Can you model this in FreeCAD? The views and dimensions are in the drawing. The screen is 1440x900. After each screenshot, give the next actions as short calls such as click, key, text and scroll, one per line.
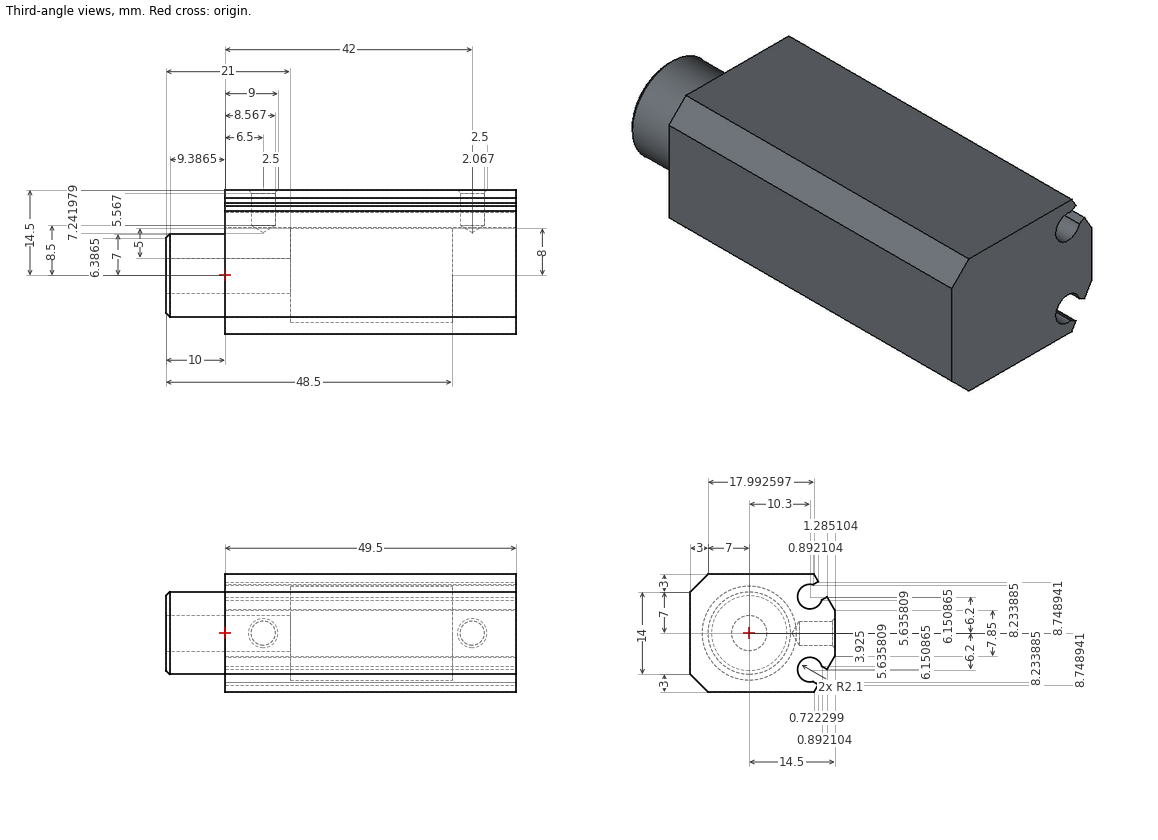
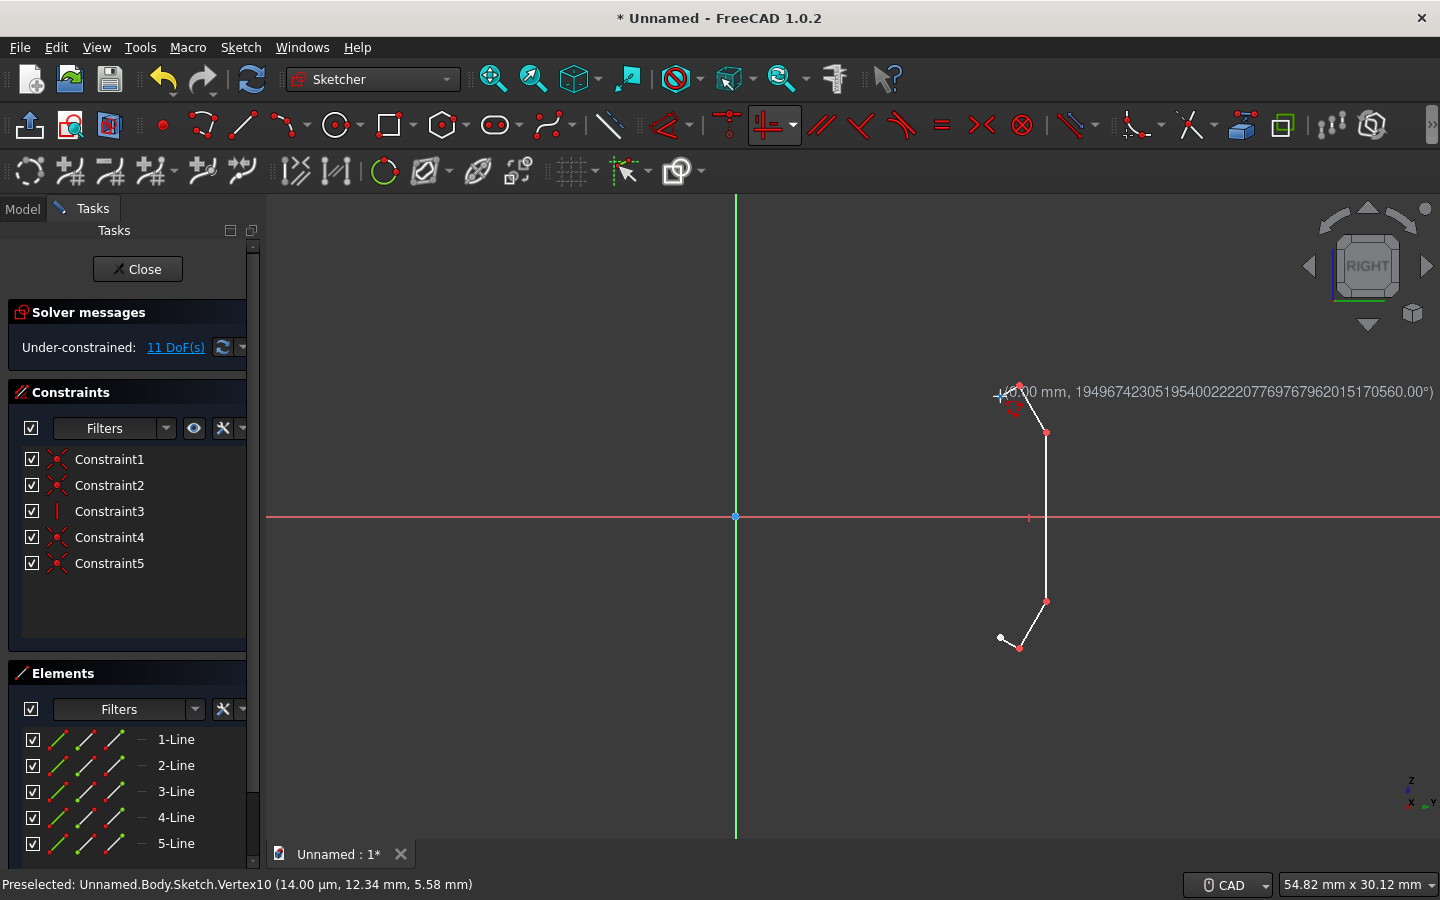
click(968, 340)
click(987, 329)
click(971, 302)
click(586, 302)
click(522, 367)
click(522, 666)
click(586, 731)
click(971, 731)
click(987, 704)
click(968, 693)
right_click(968, 693)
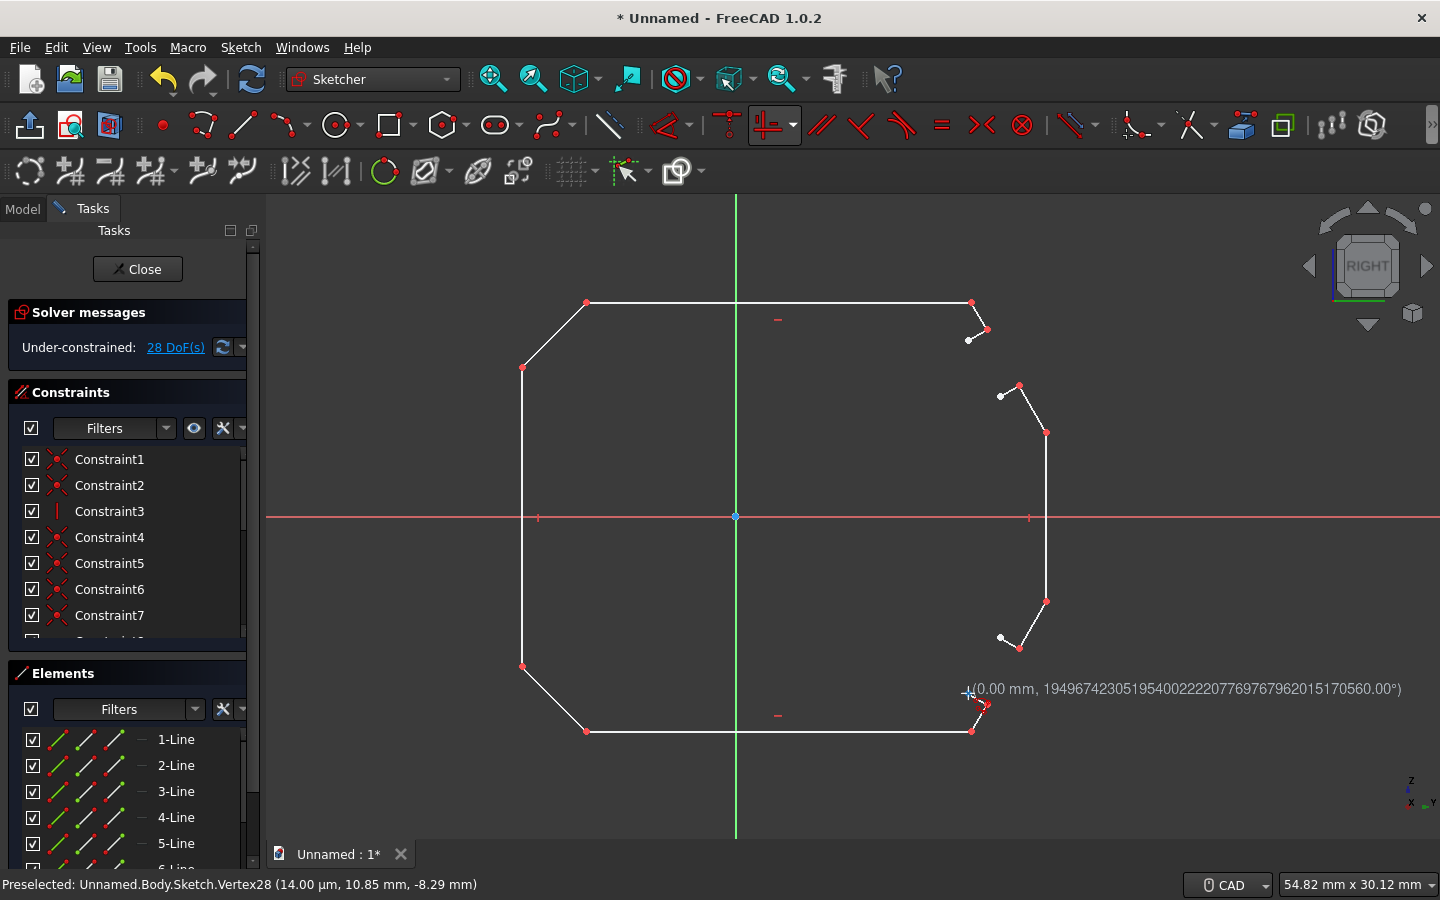
key(g)
key(3)
key(a)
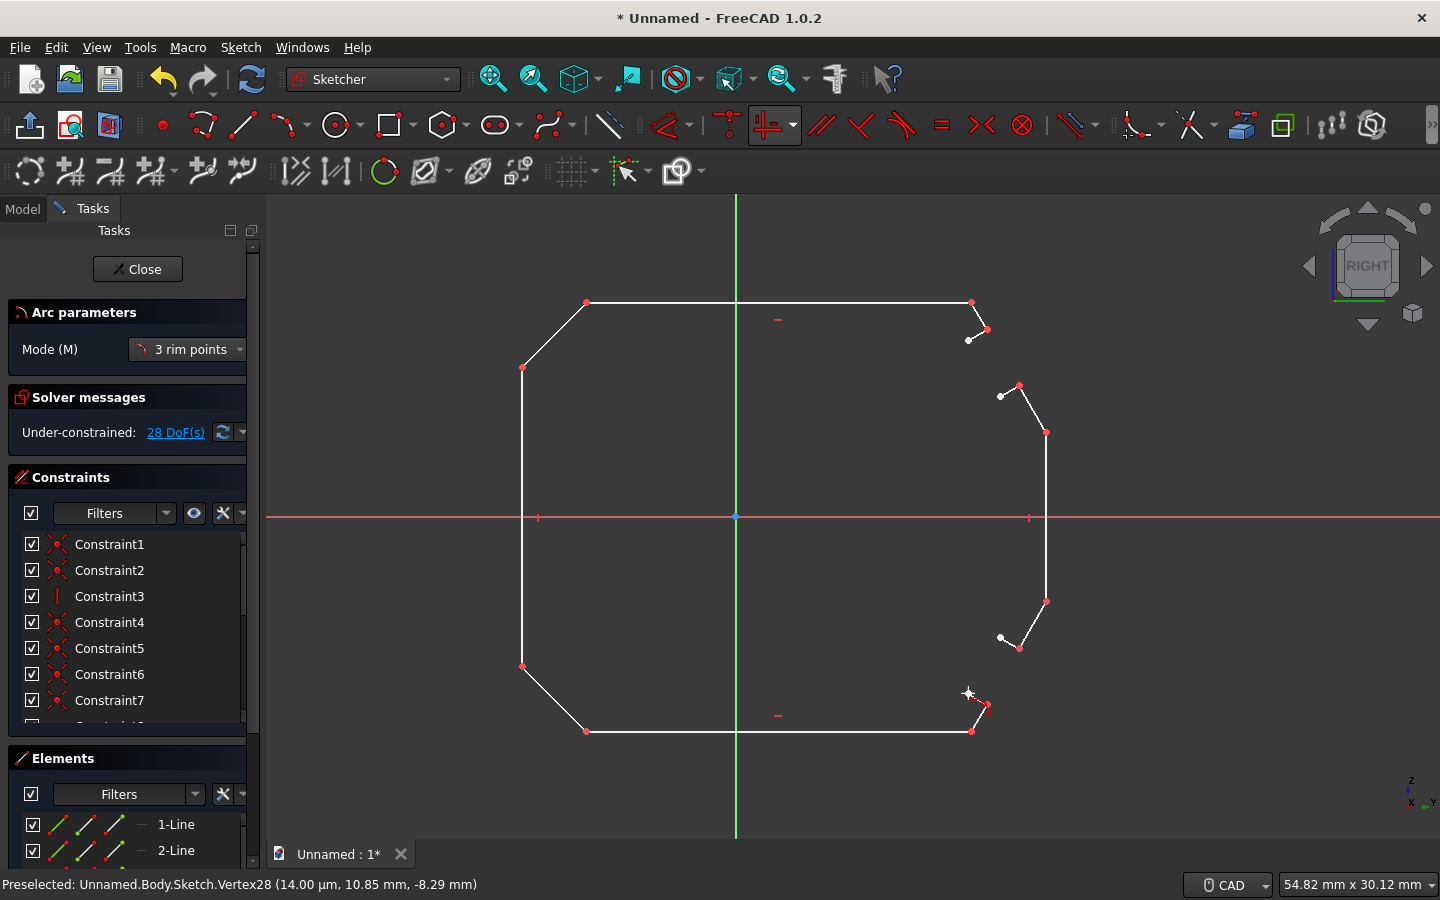
scroll(1000, 396, up, 2)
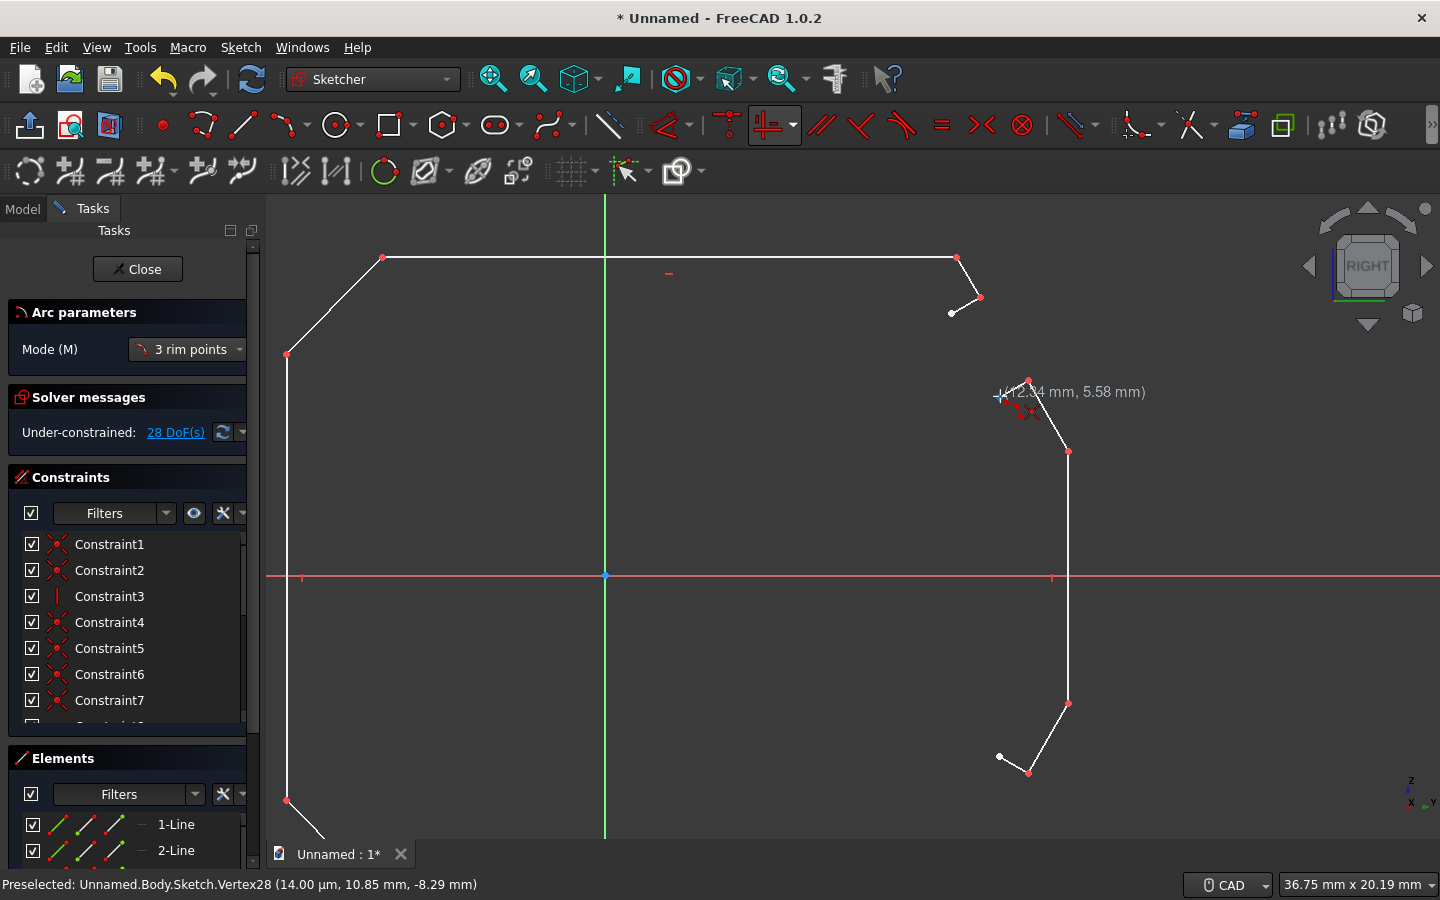
click(1000, 397)
click(952, 314)
click(876, 411)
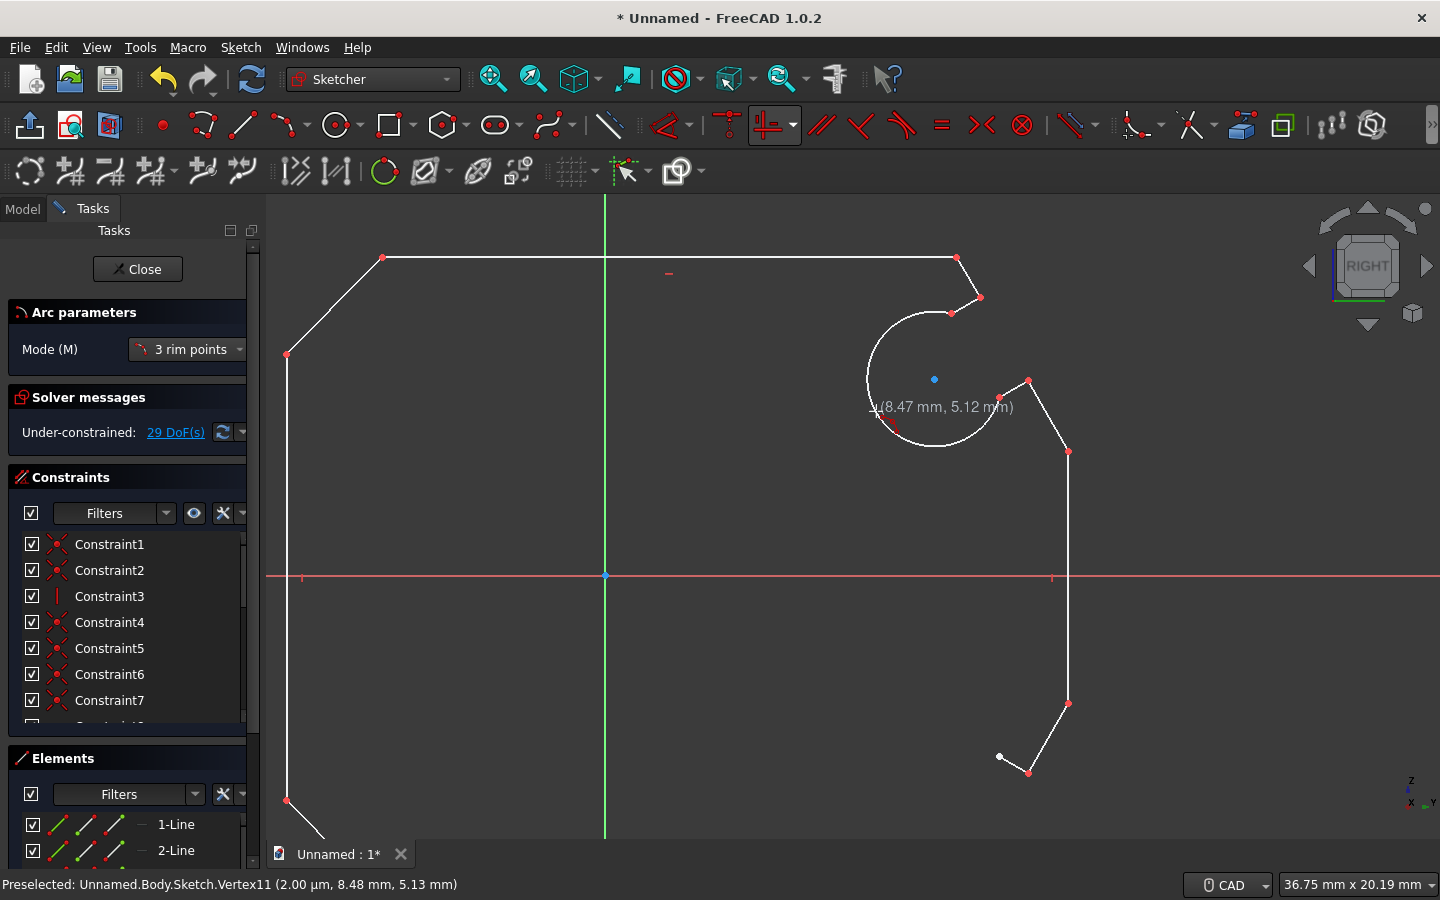
scroll(1002, 396, down, 2)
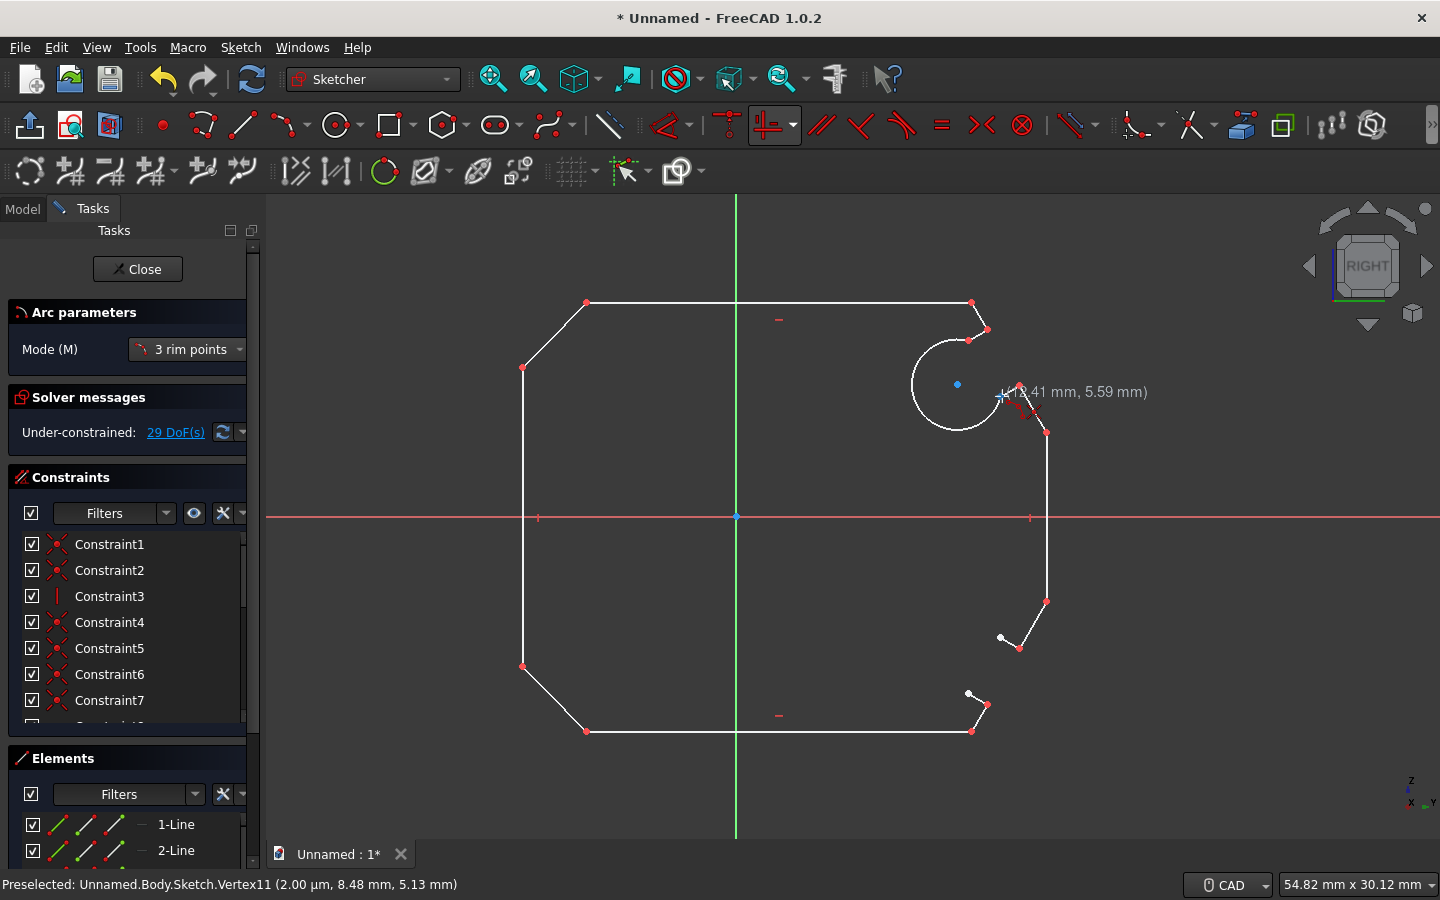
scroll(968, 693, up, 2)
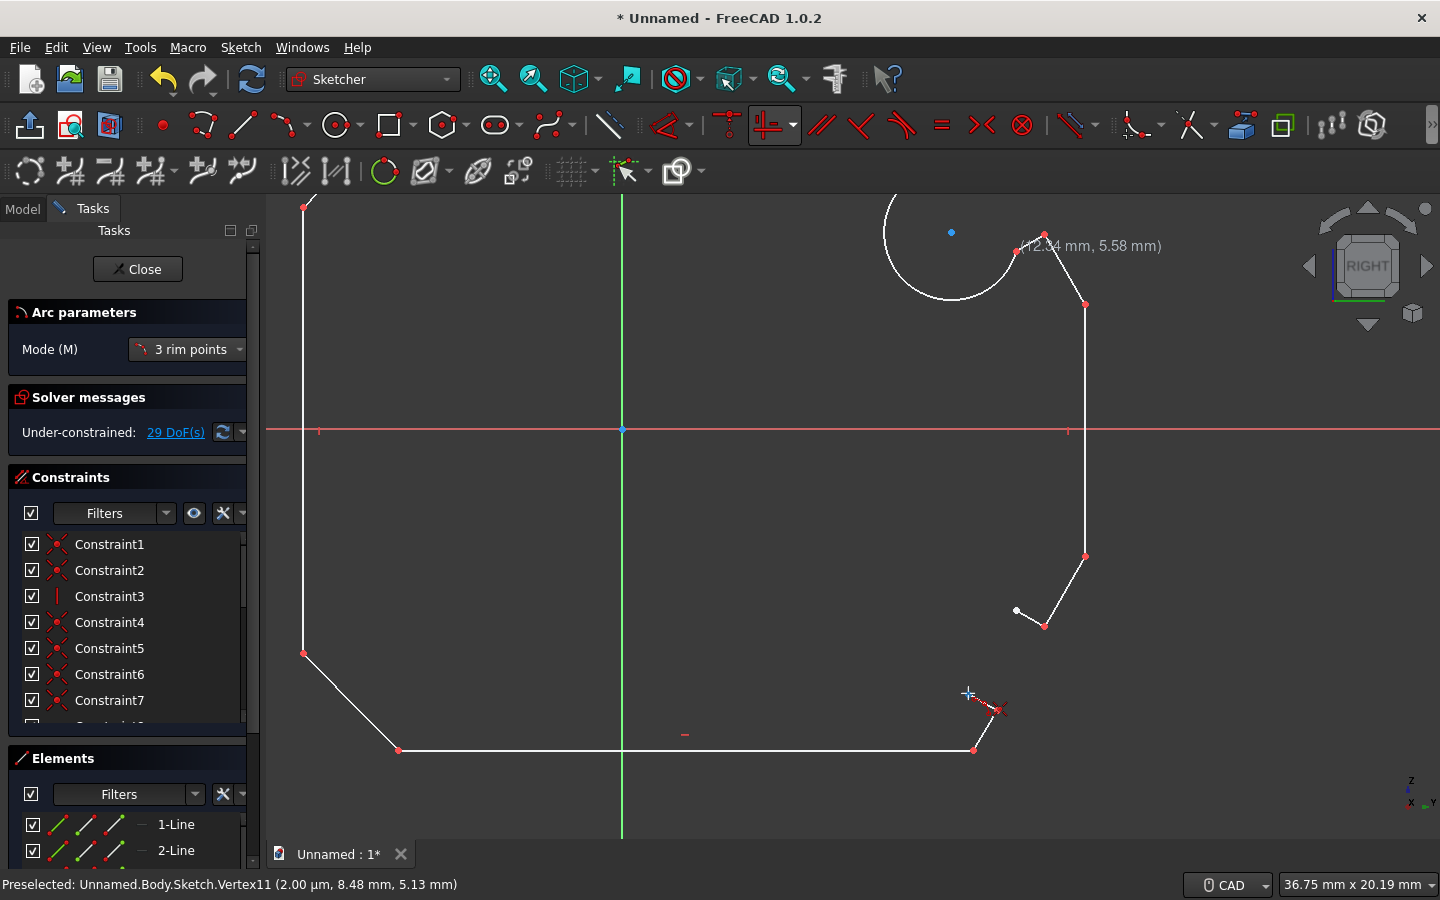
click(969, 694)
click(1016, 611)
click(893, 594)
key(Escape)